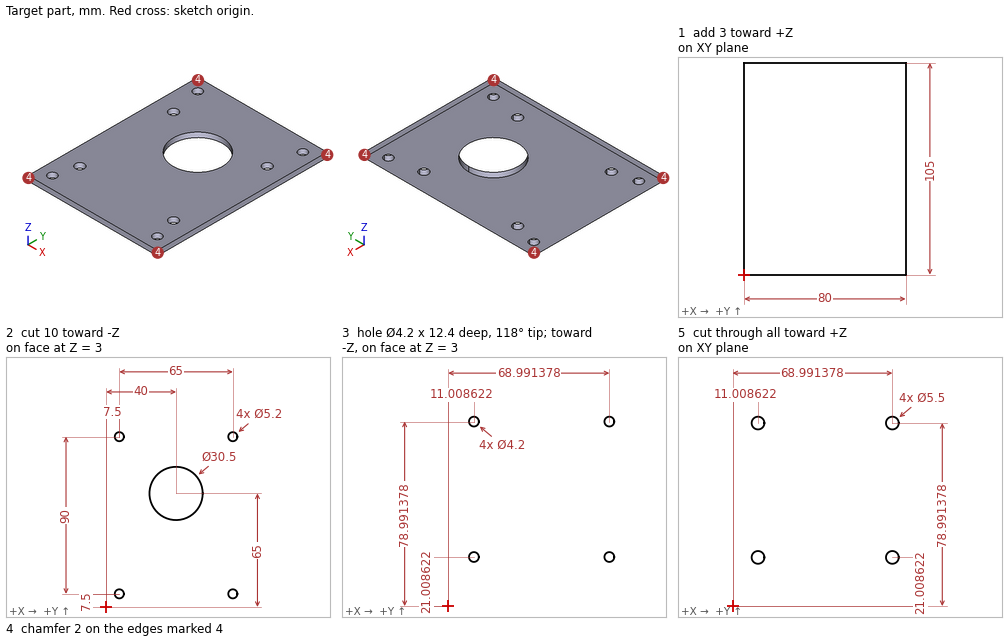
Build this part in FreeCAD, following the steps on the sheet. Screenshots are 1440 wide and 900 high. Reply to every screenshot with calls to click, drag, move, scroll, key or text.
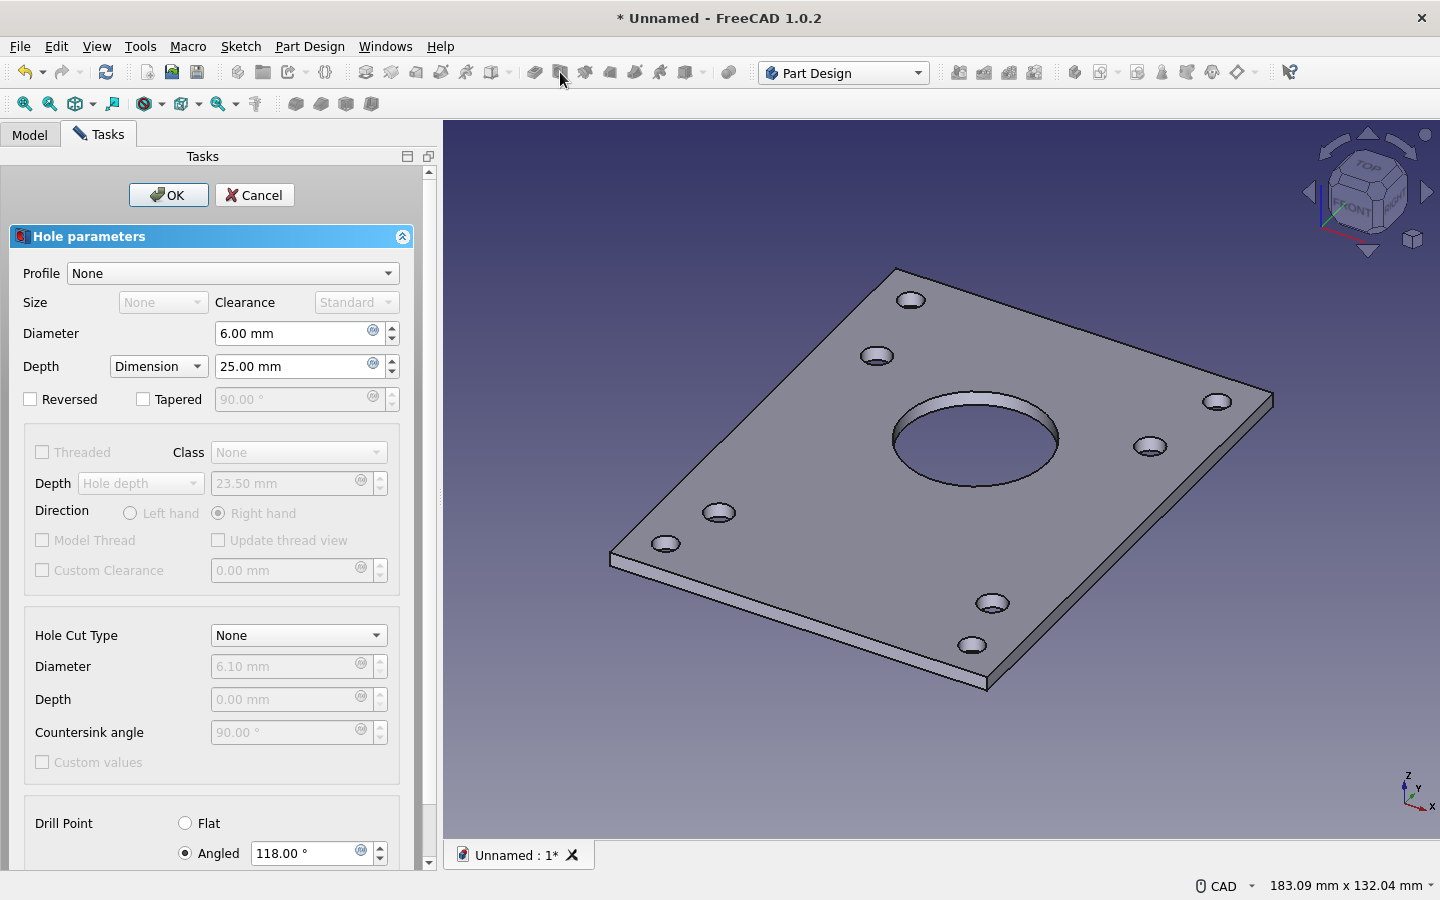
triple_click(300, 334)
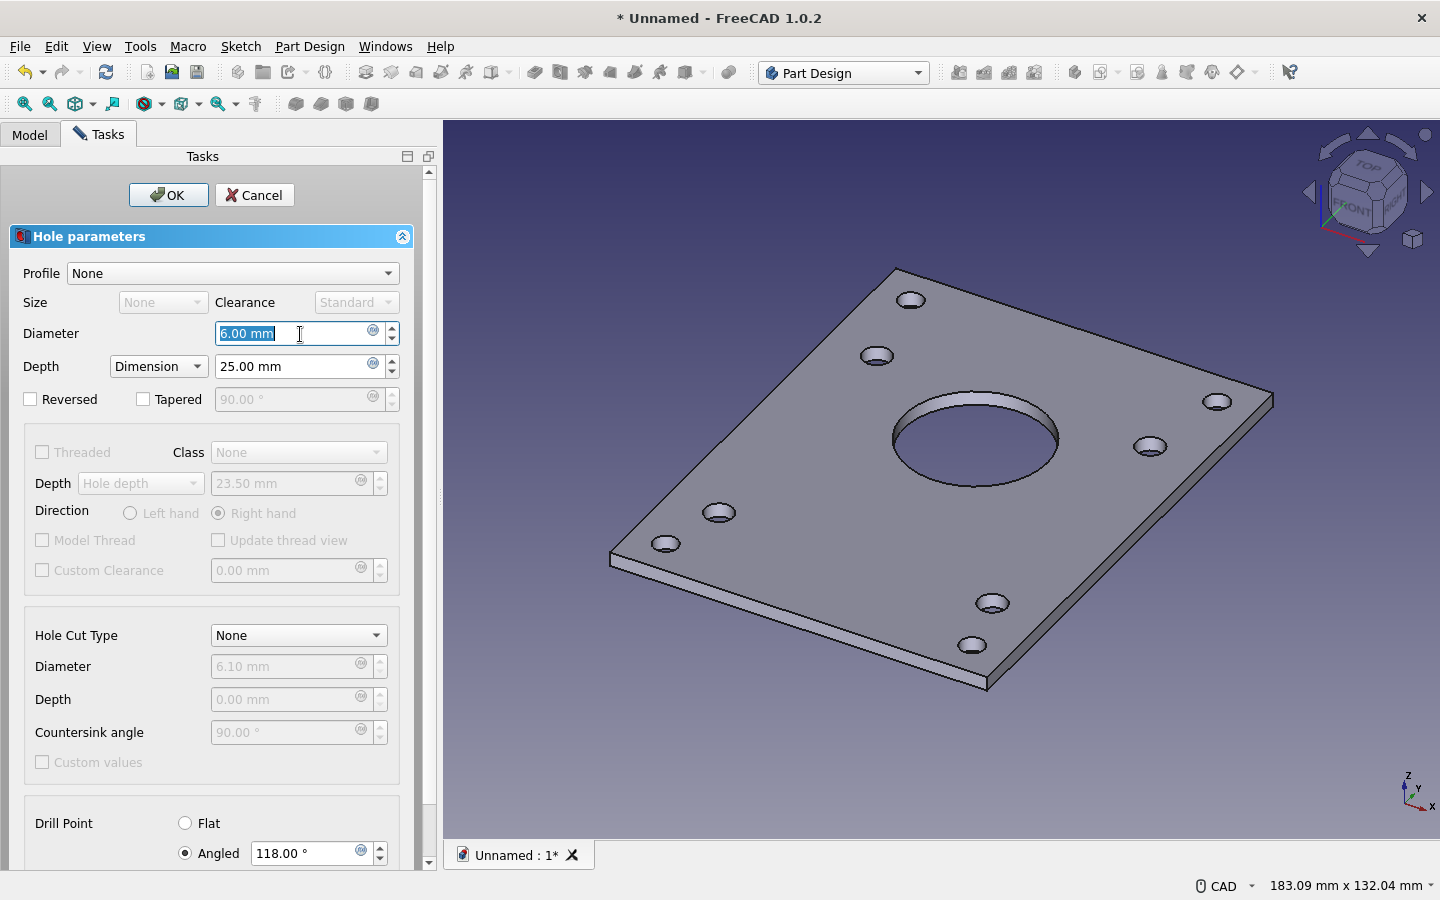
text(4.2)
key(Tab)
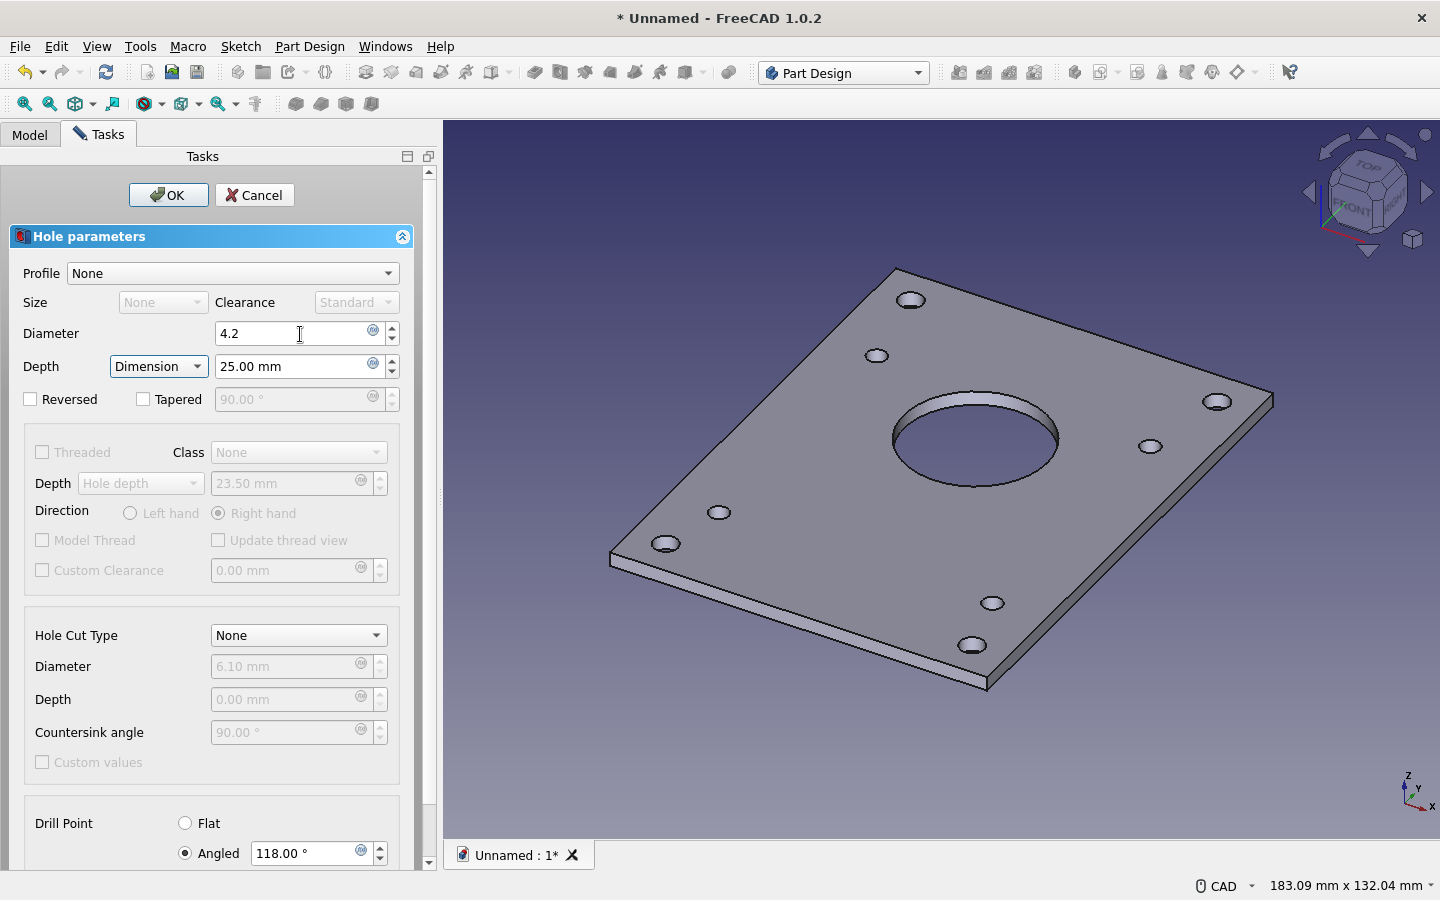
triple_click(300, 366)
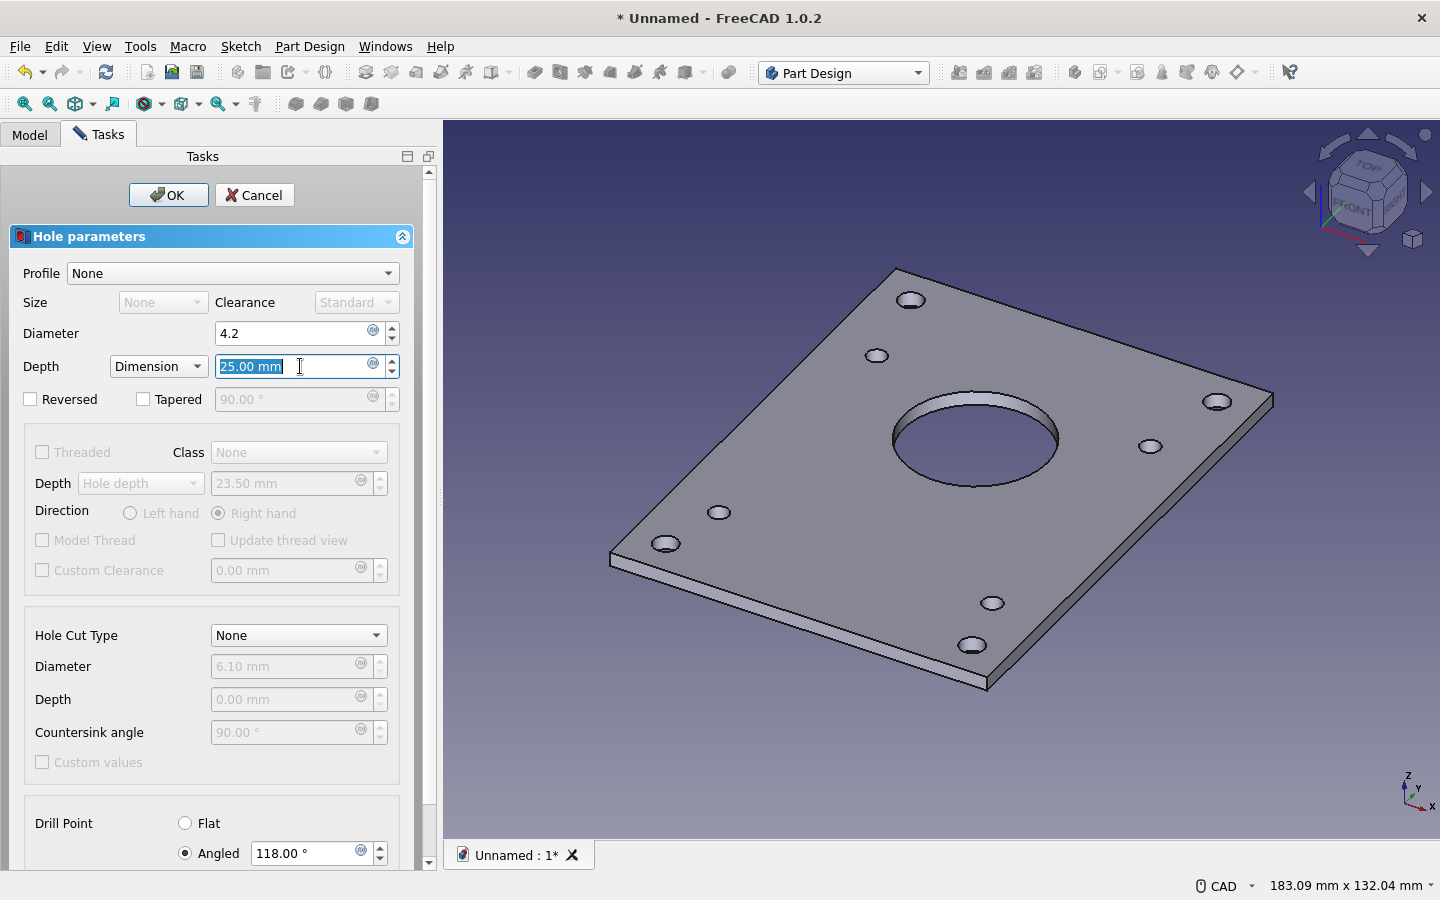
text(12.4)
key(Tab)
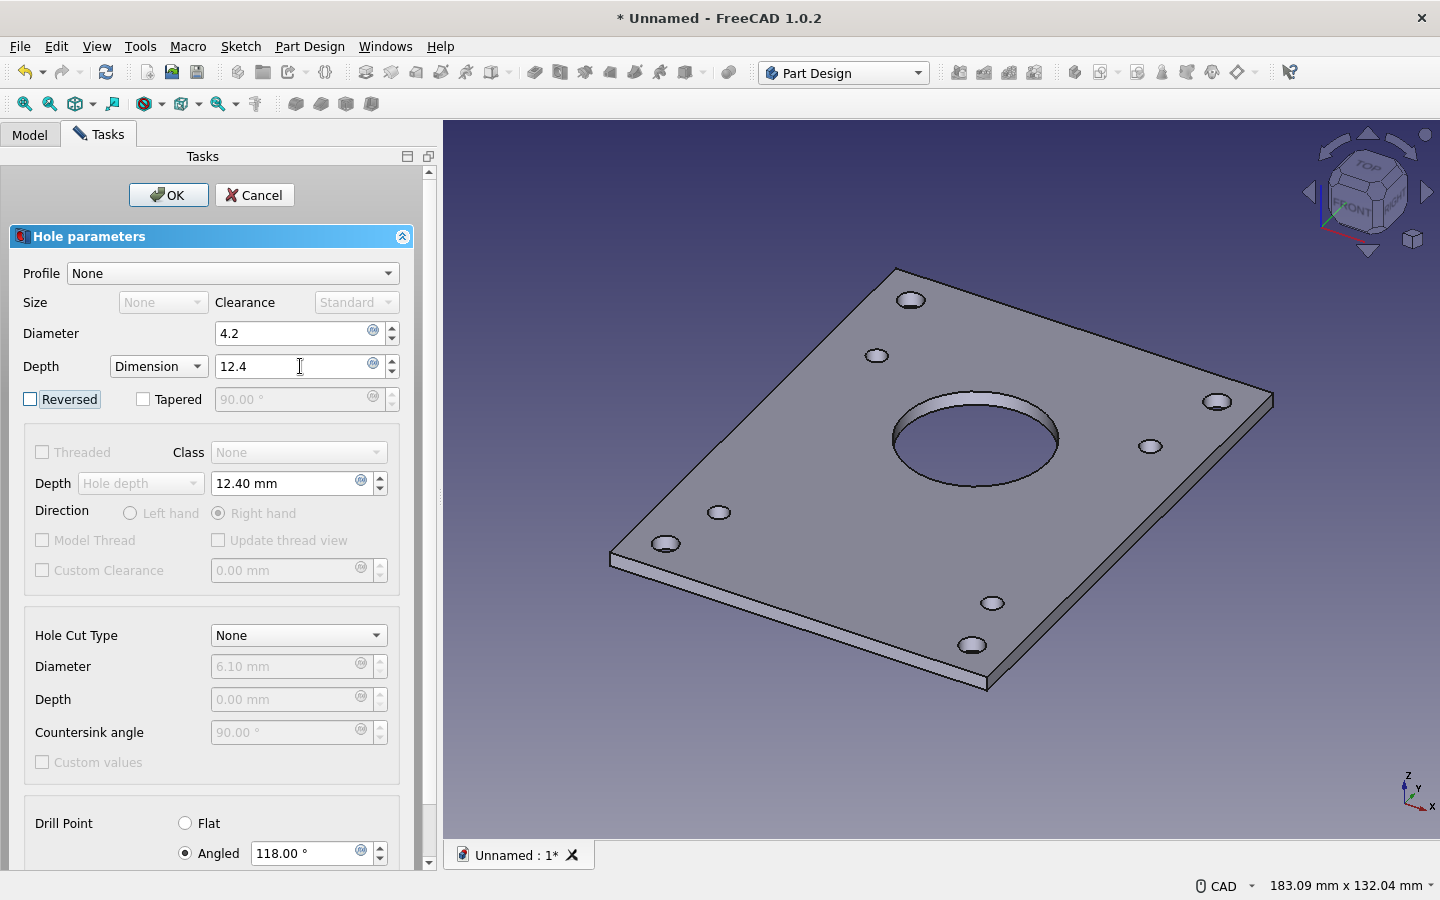
click(169, 195)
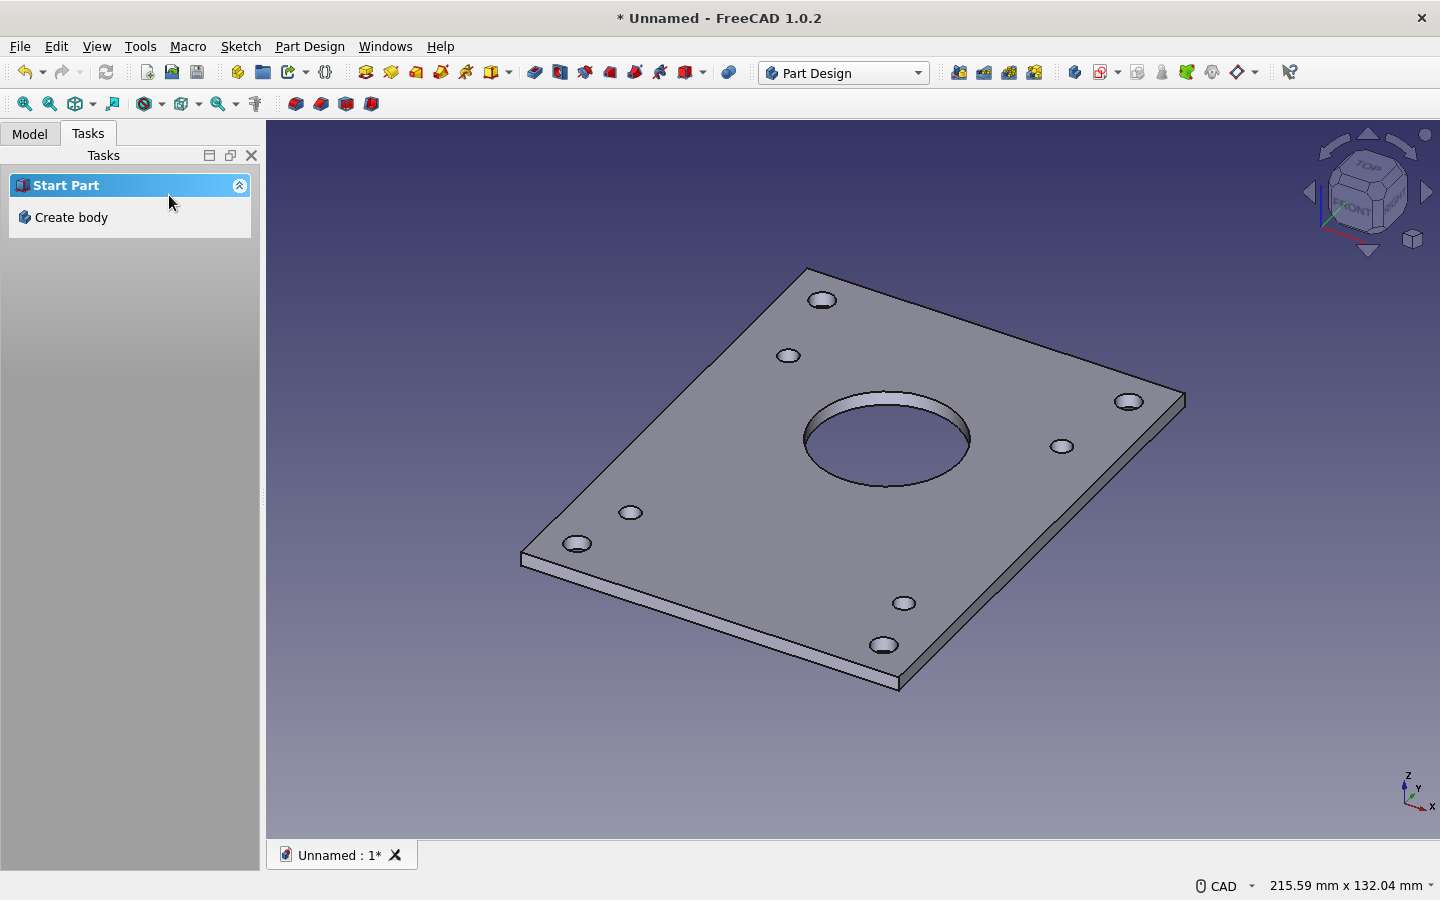
click(899, 683)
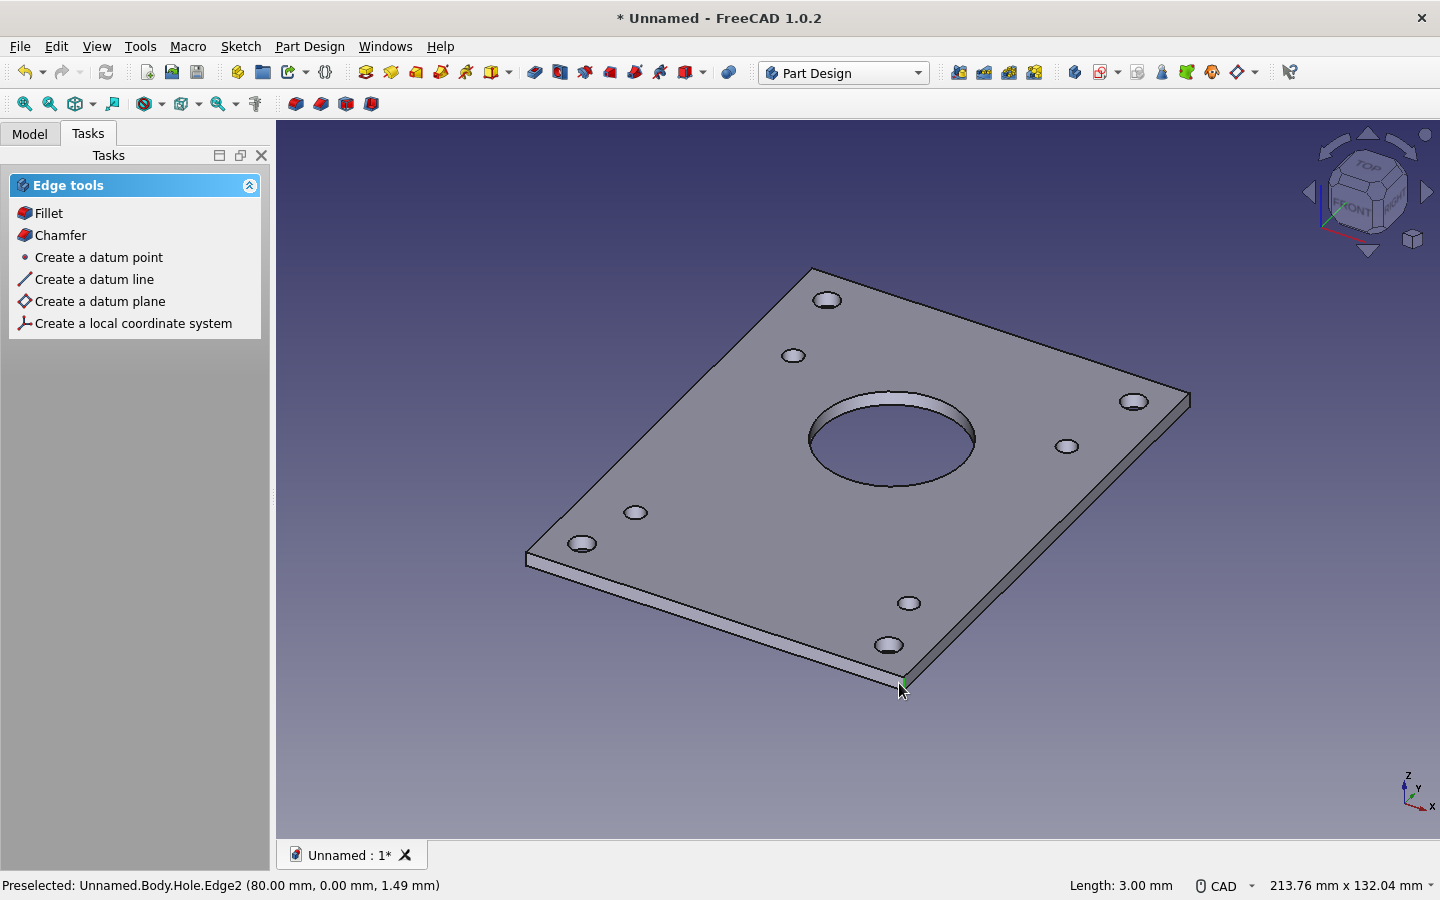
scroll(812, 274, up, 5)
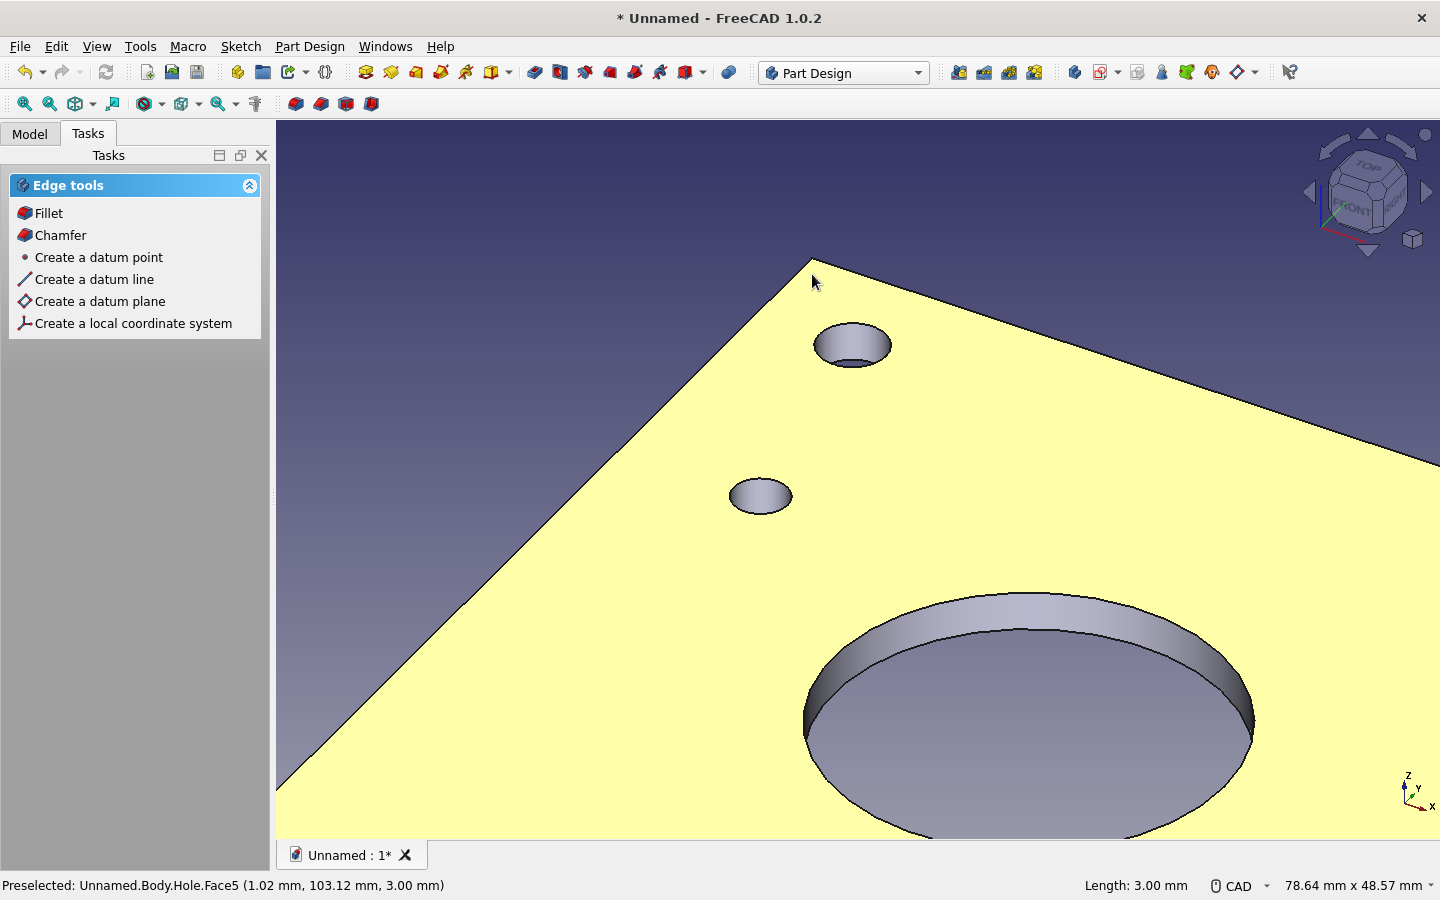
click(25, 104)